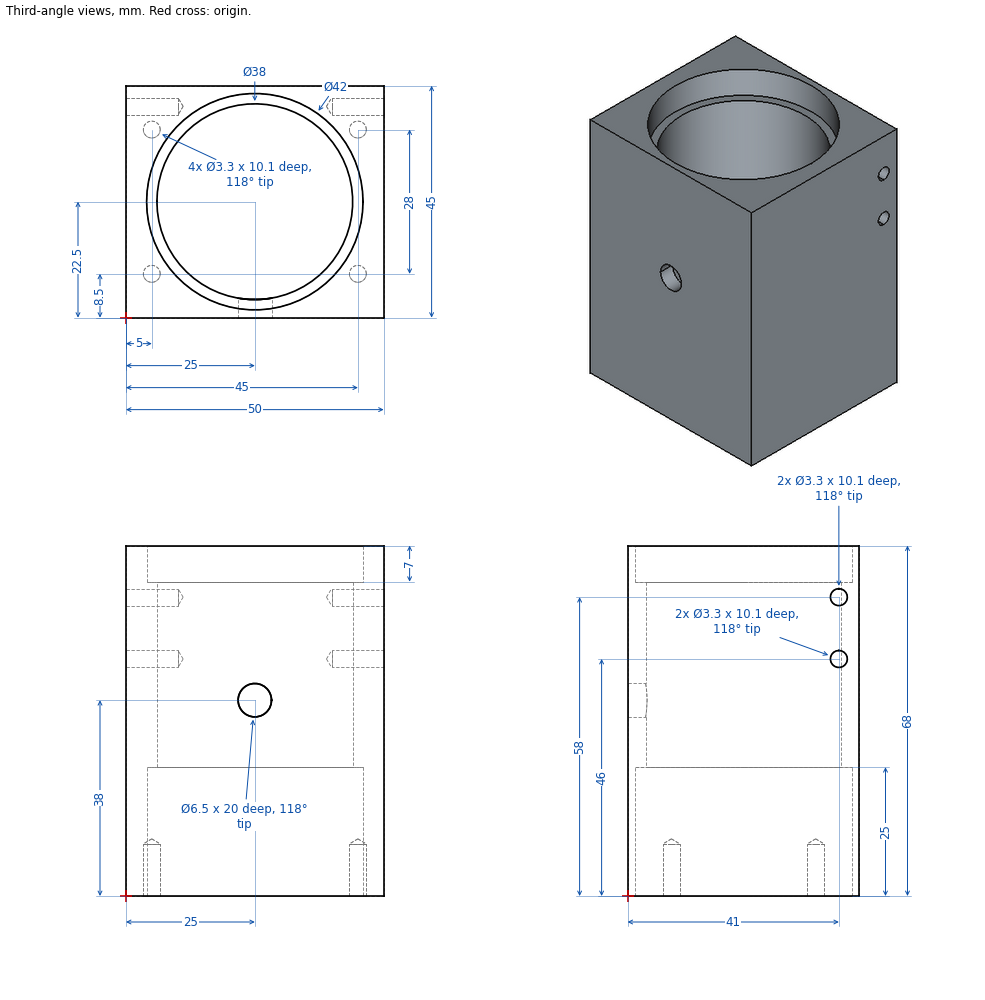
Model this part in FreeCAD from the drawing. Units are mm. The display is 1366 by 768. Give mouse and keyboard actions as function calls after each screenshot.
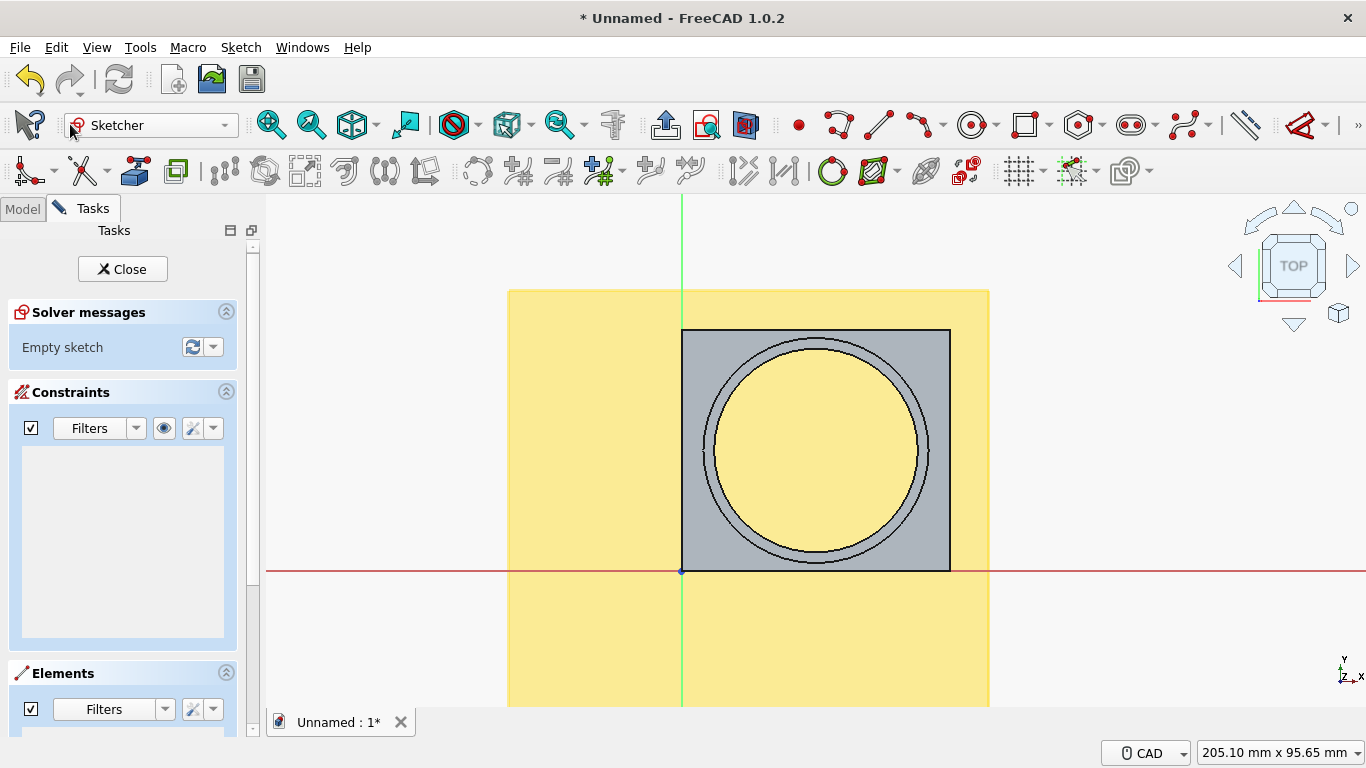
click(746, 126)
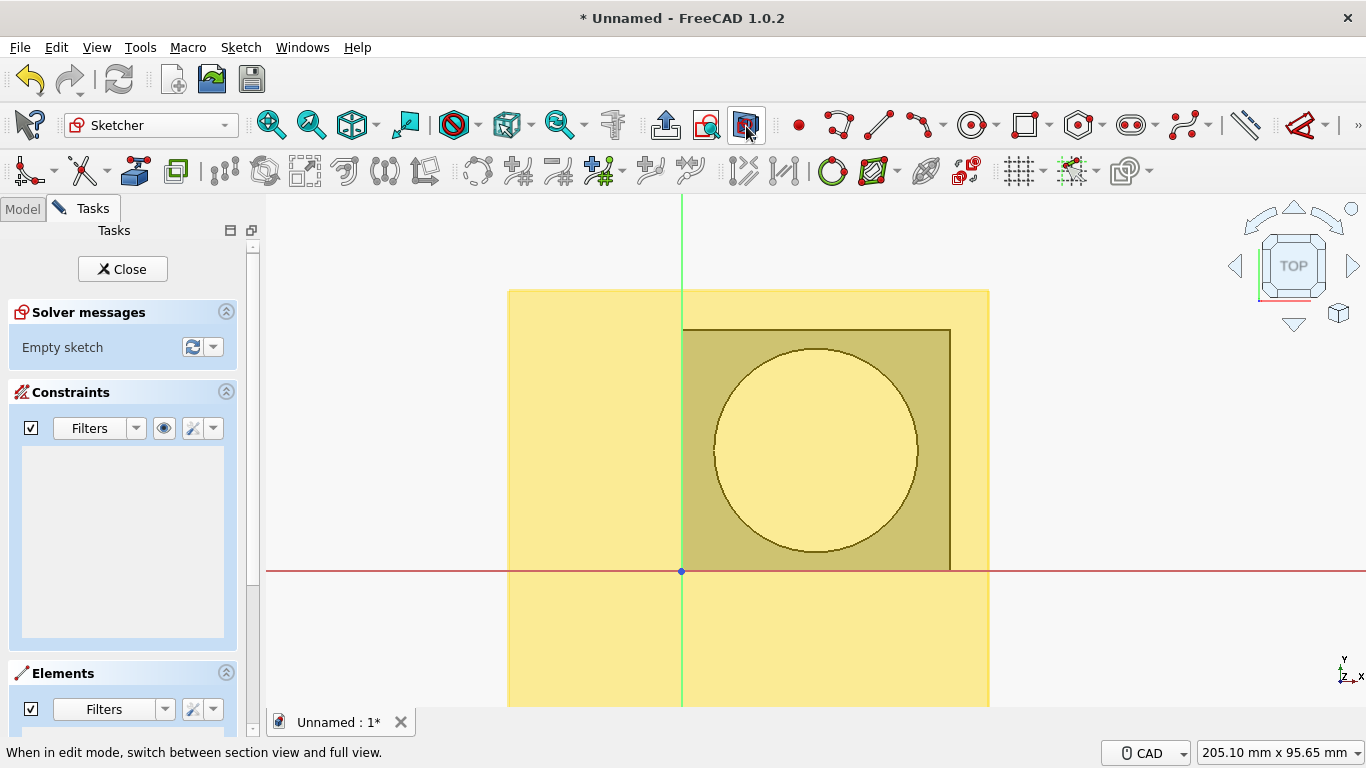
scroll(923, 463, up, 2)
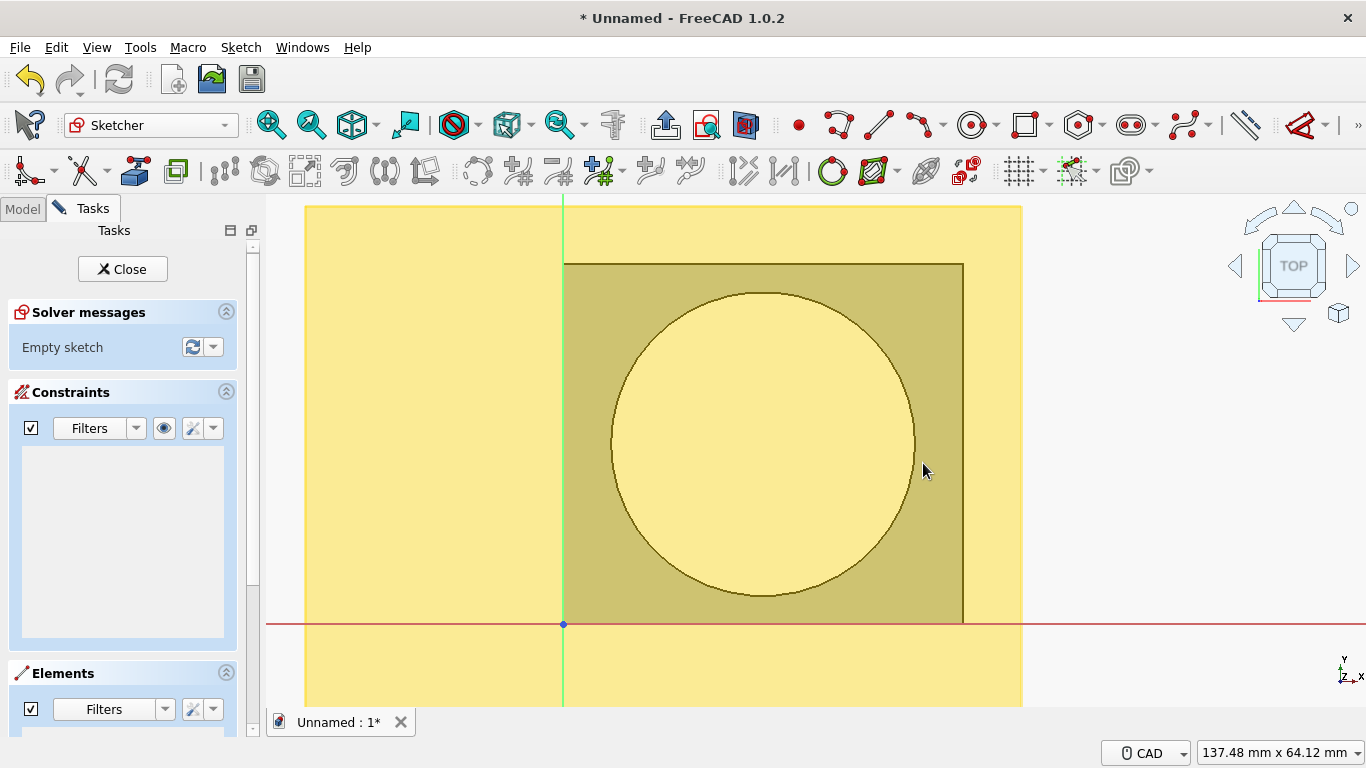
click(972, 126)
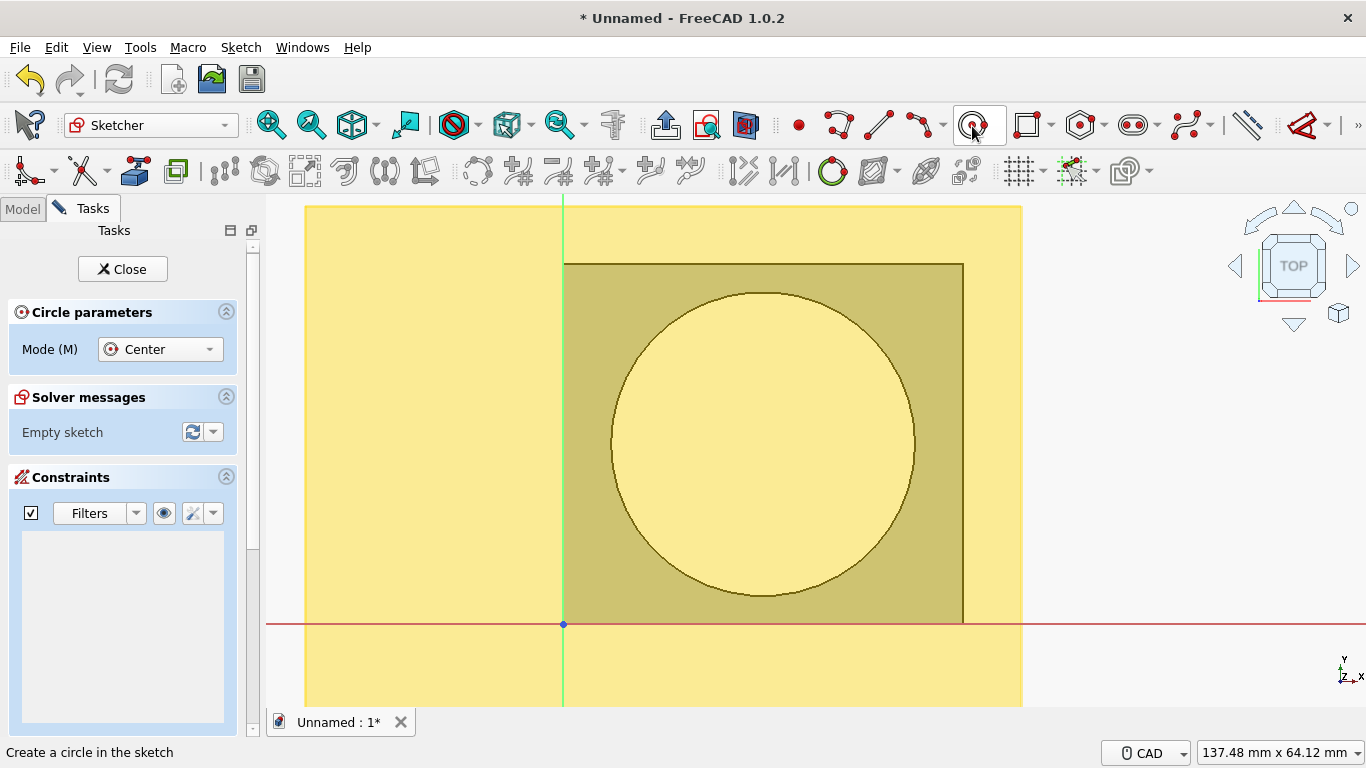
click(763, 444)
move(882, 325)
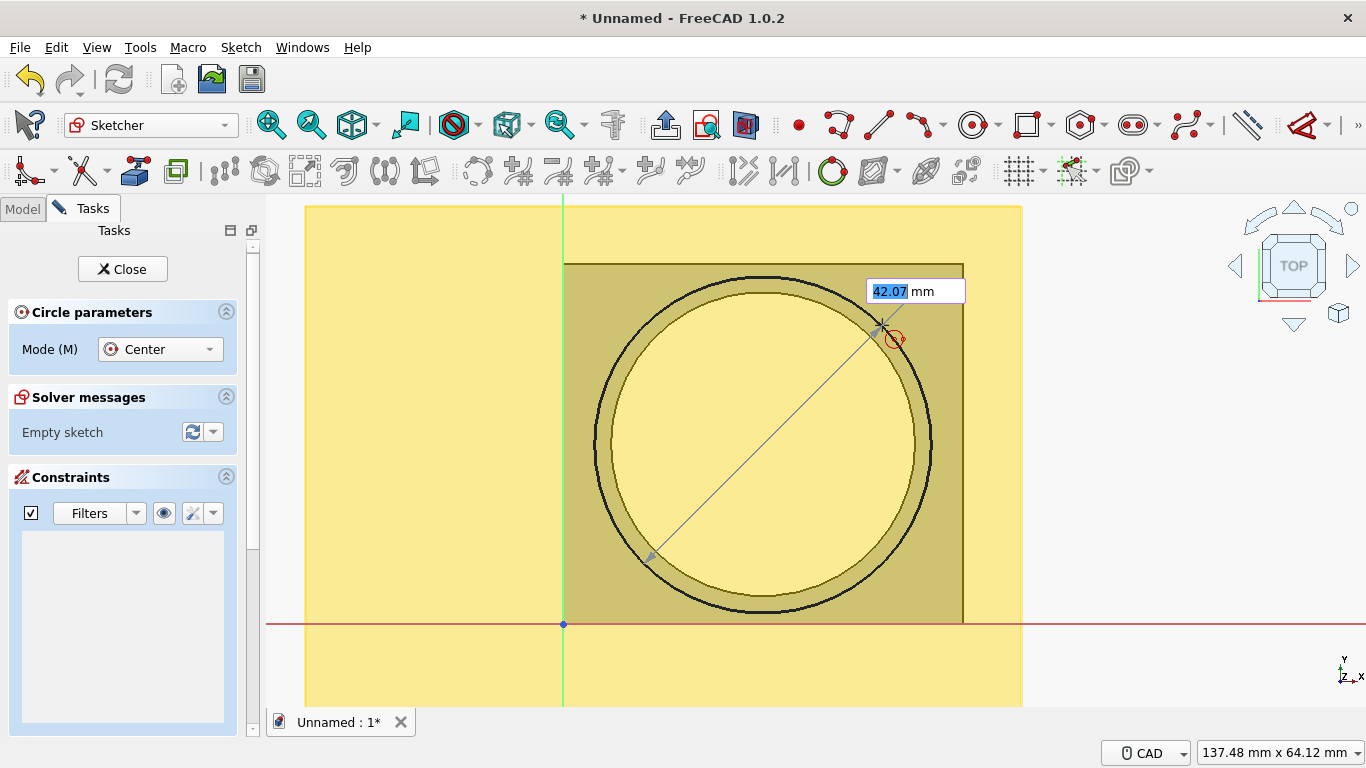
text(42)
key(Return)
key(Escape)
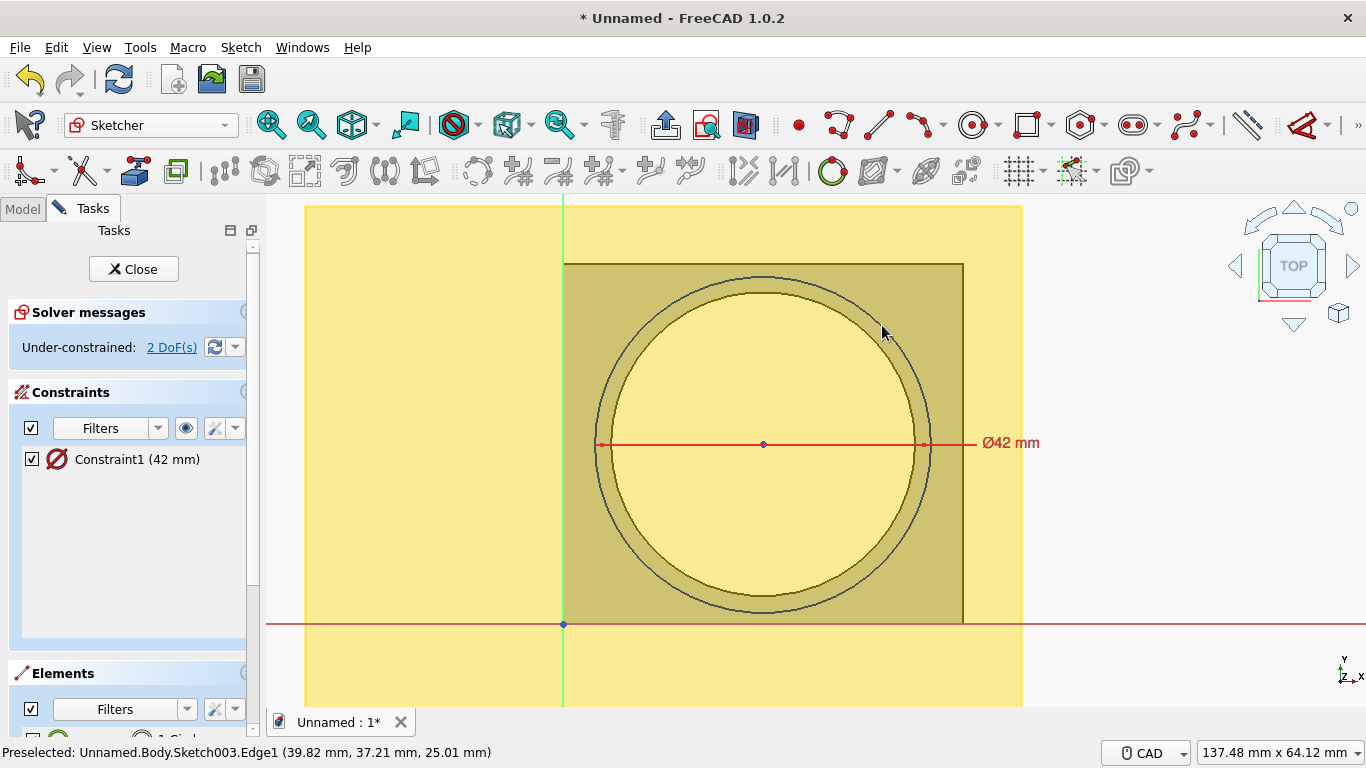
click(1302, 126)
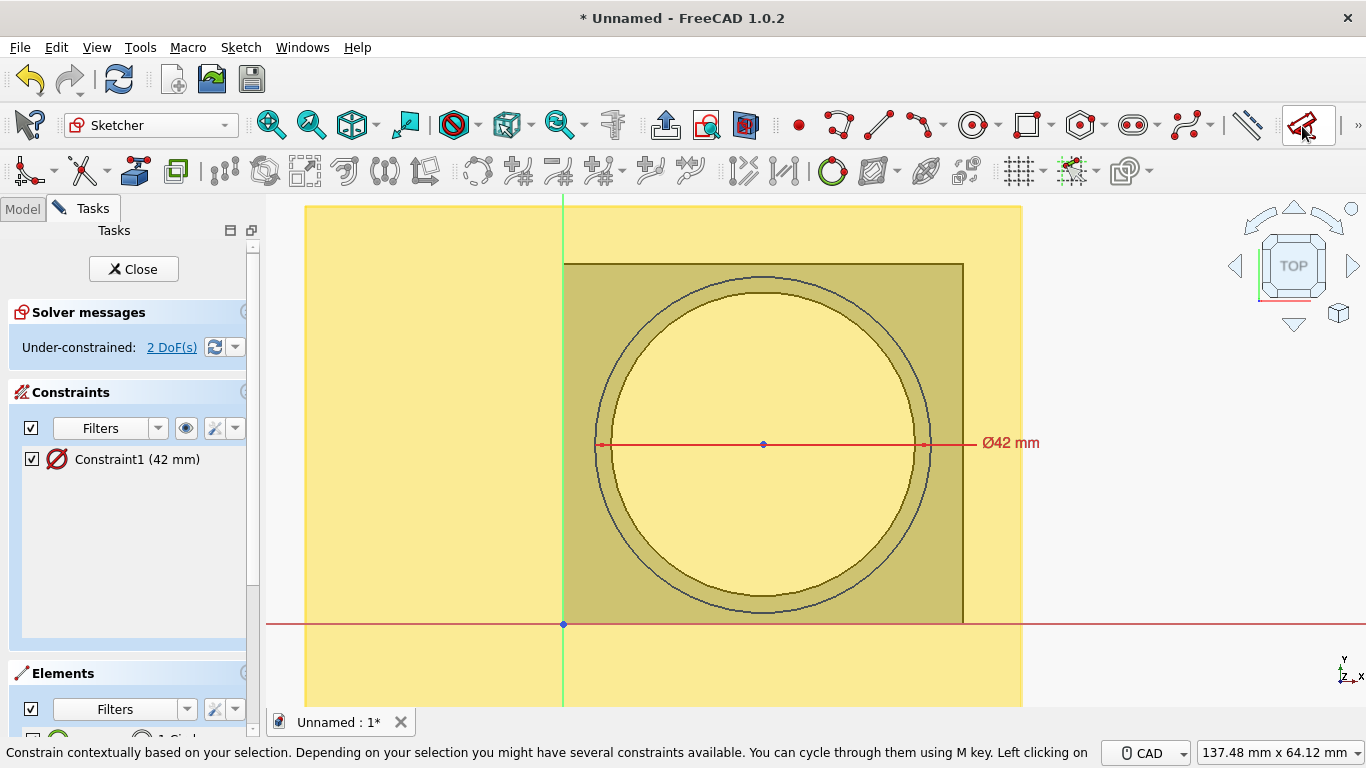
click(763, 445)
click(663, 658)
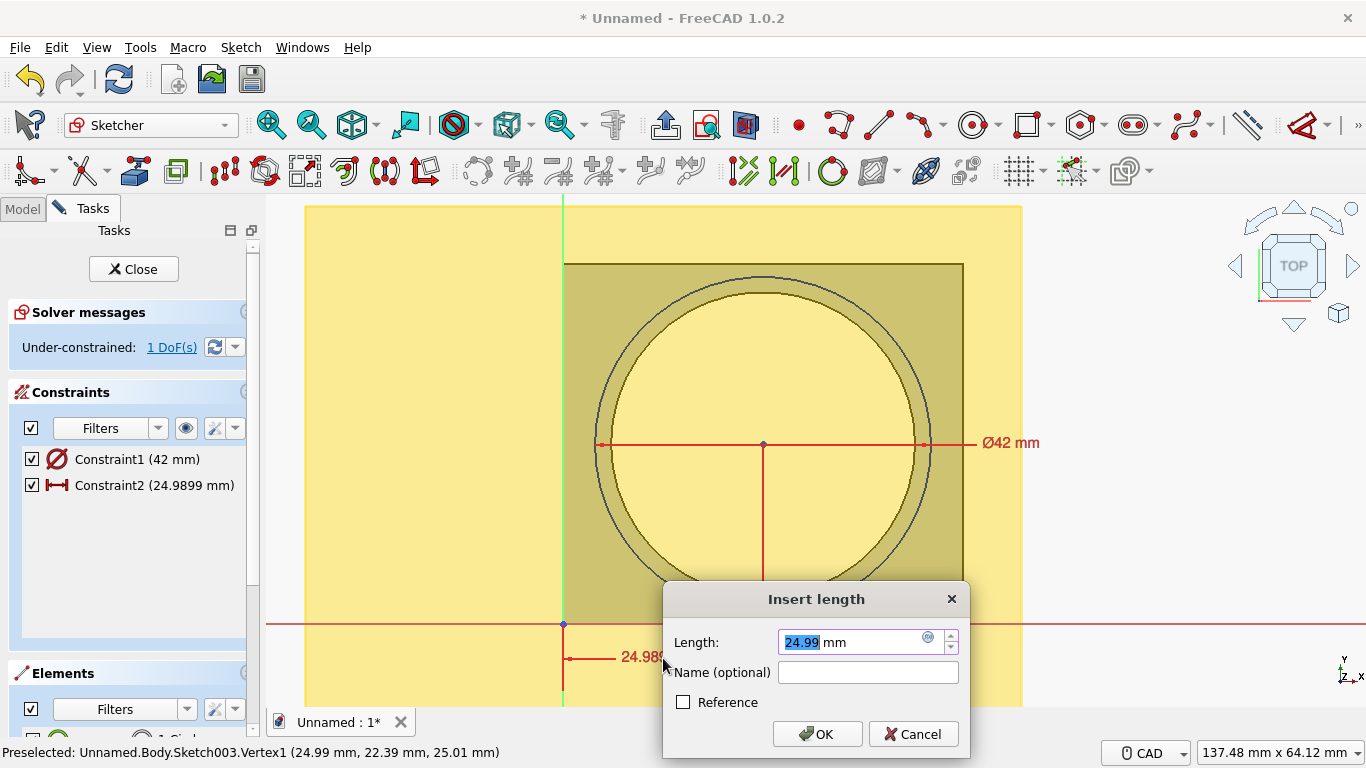
text(25)
key(Return)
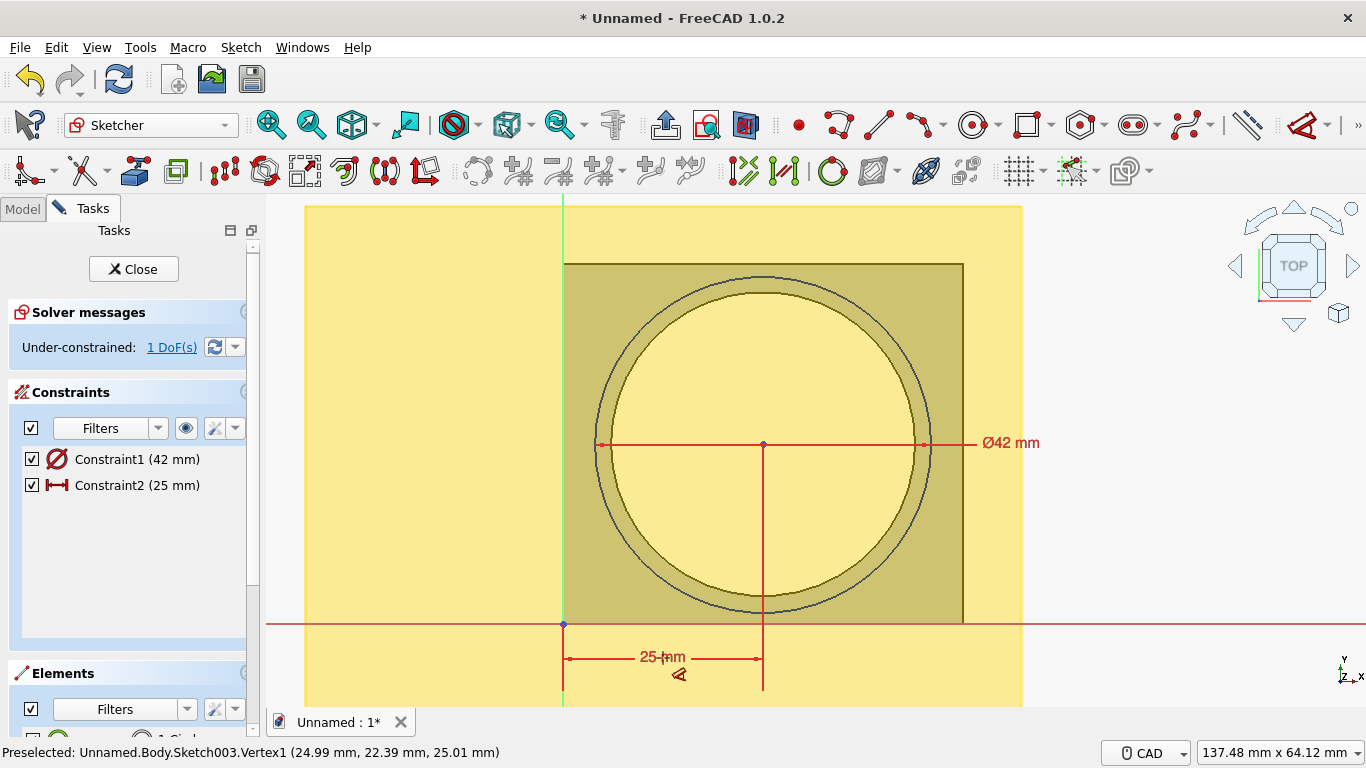
click(763, 445)
click(529, 535)